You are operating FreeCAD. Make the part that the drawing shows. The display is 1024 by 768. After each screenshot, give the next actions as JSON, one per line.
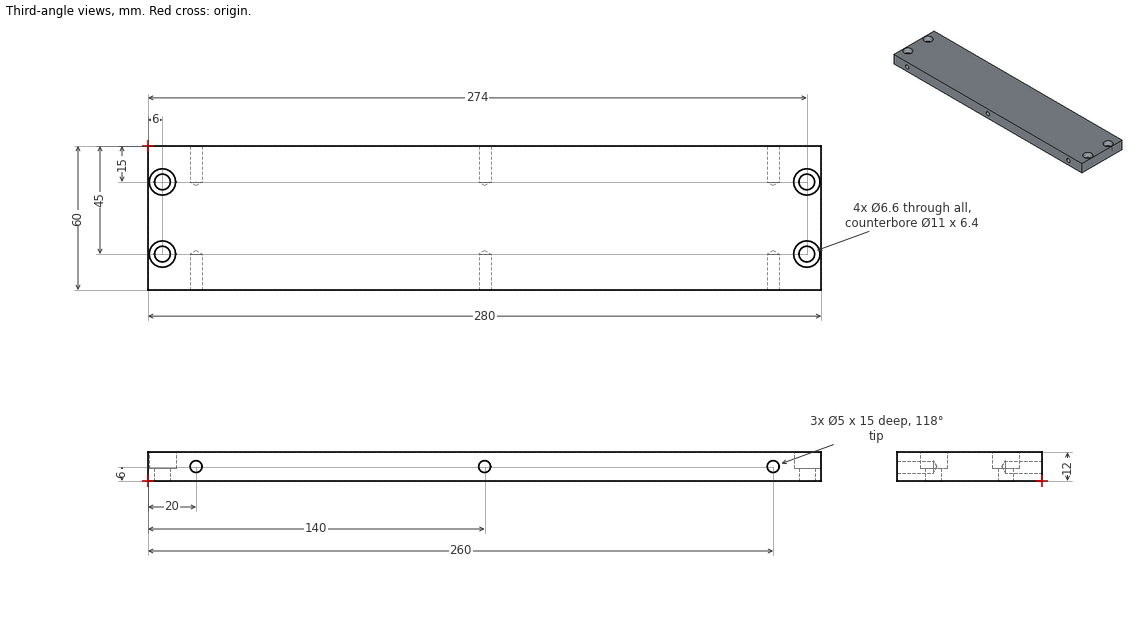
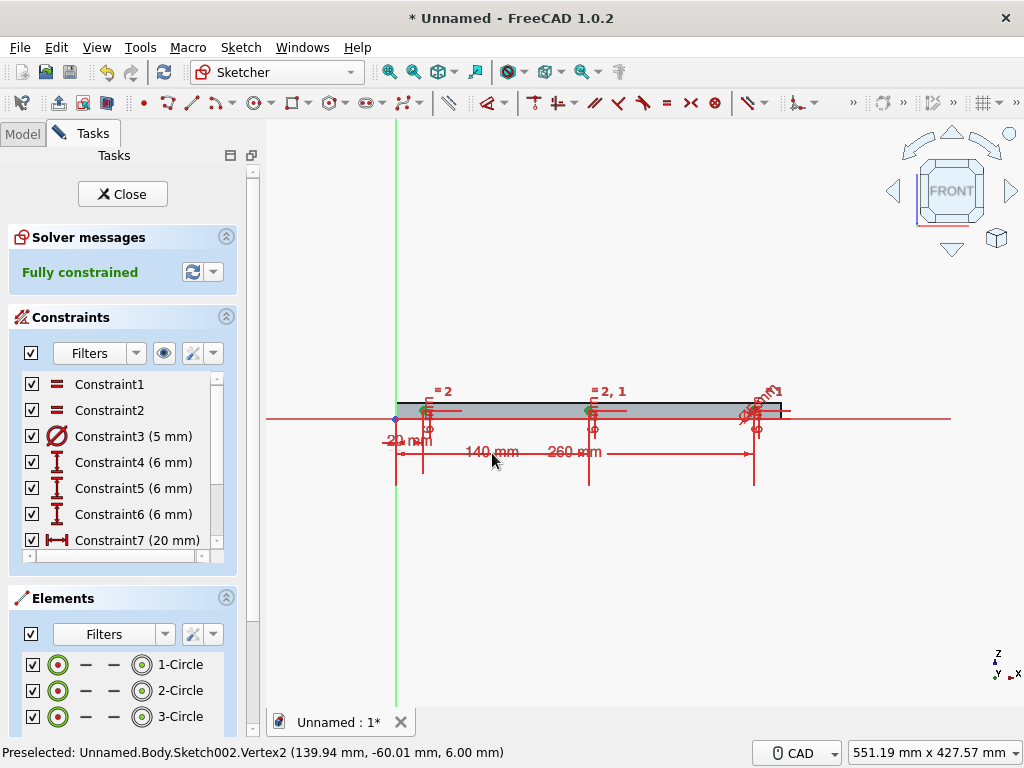
{"action": "left_click", "coordinate": [123, 194]}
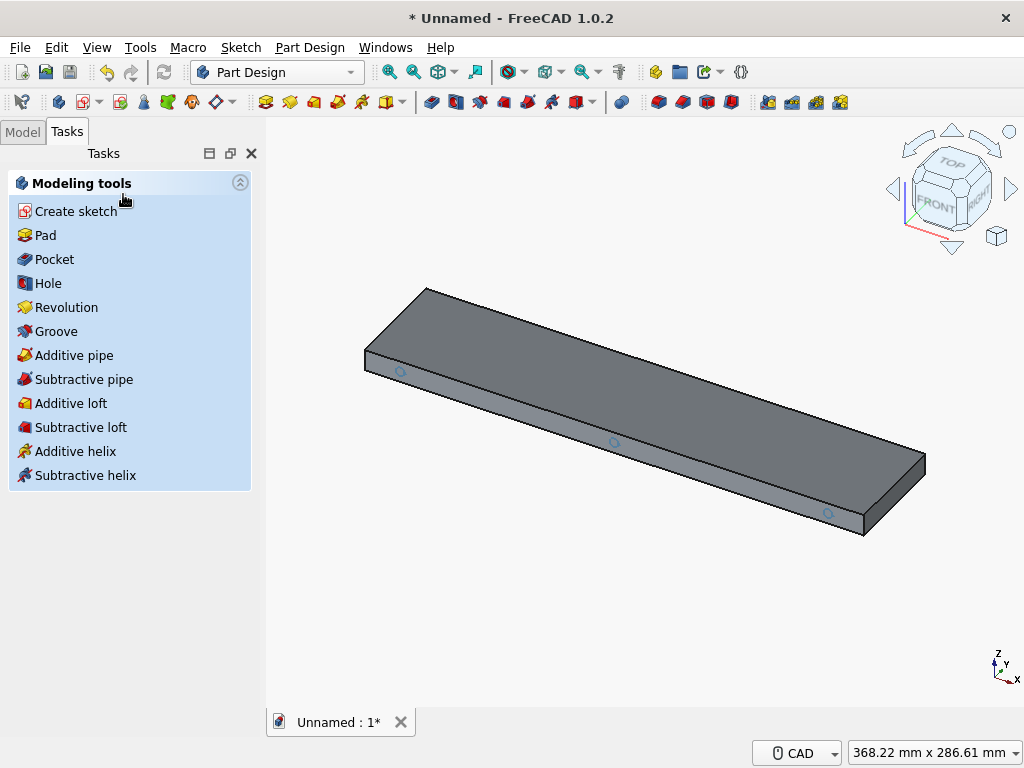
{"action": "left_click", "coordinate": [456, 102]}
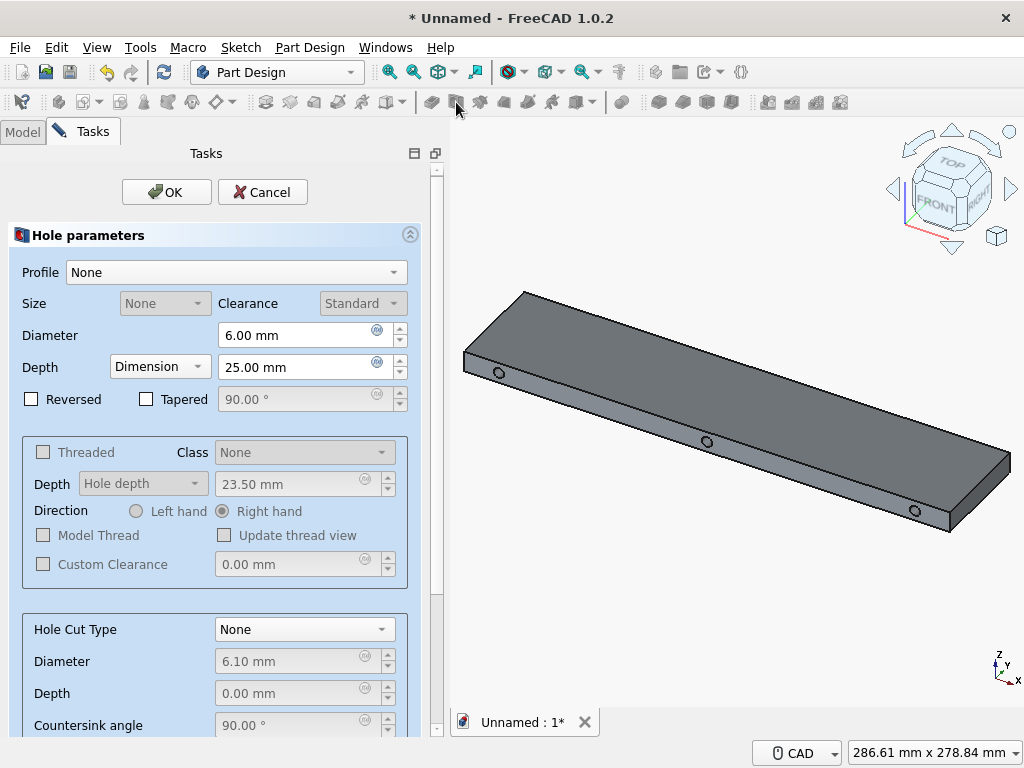
{"action": "triple_click", "coordinate": [305, 335]}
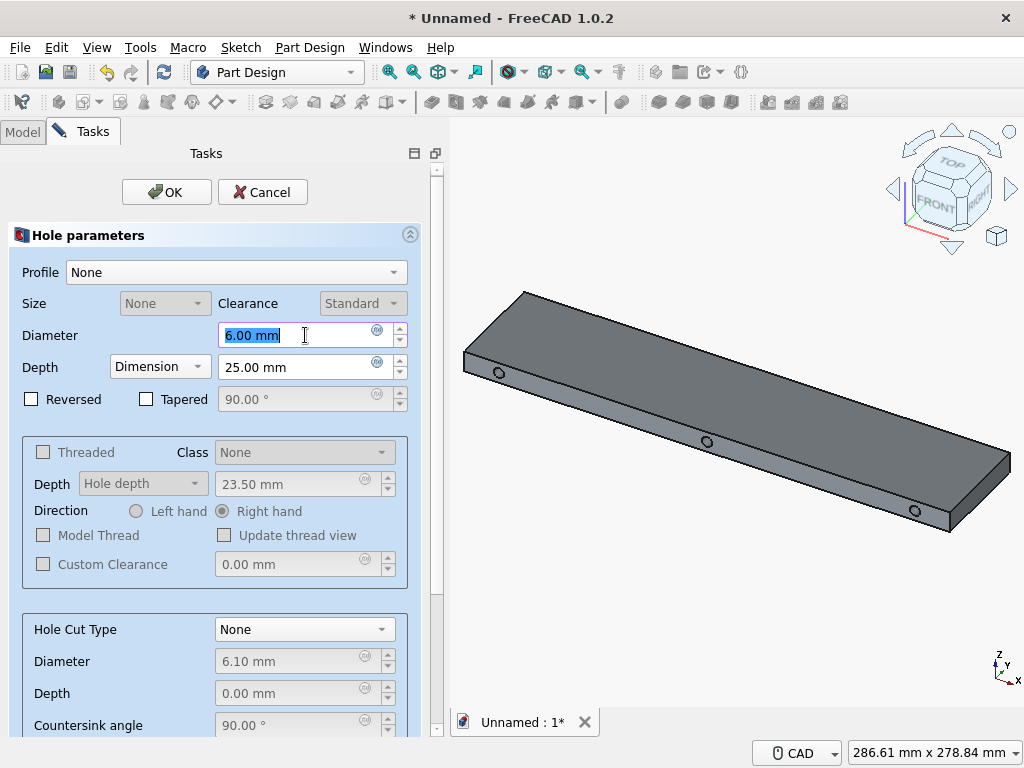
{"action": "type", "text": "5"}
{"action": "key", "text": "Tab"}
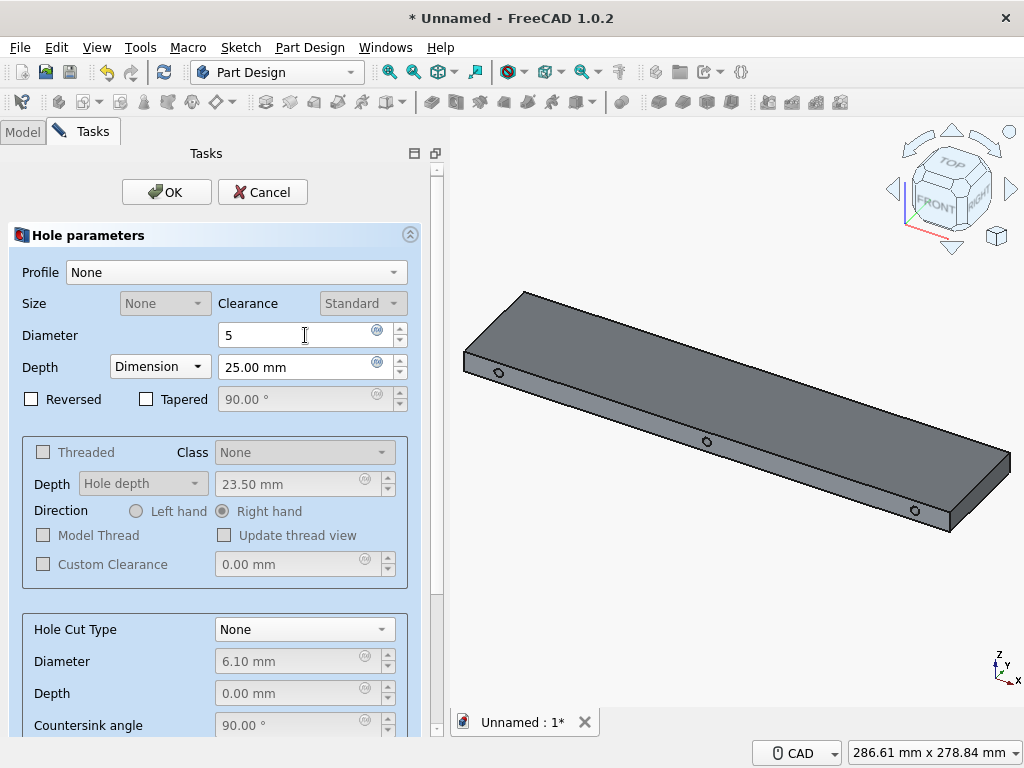
{"action": "triple_click", "coordinate": [305, 367]}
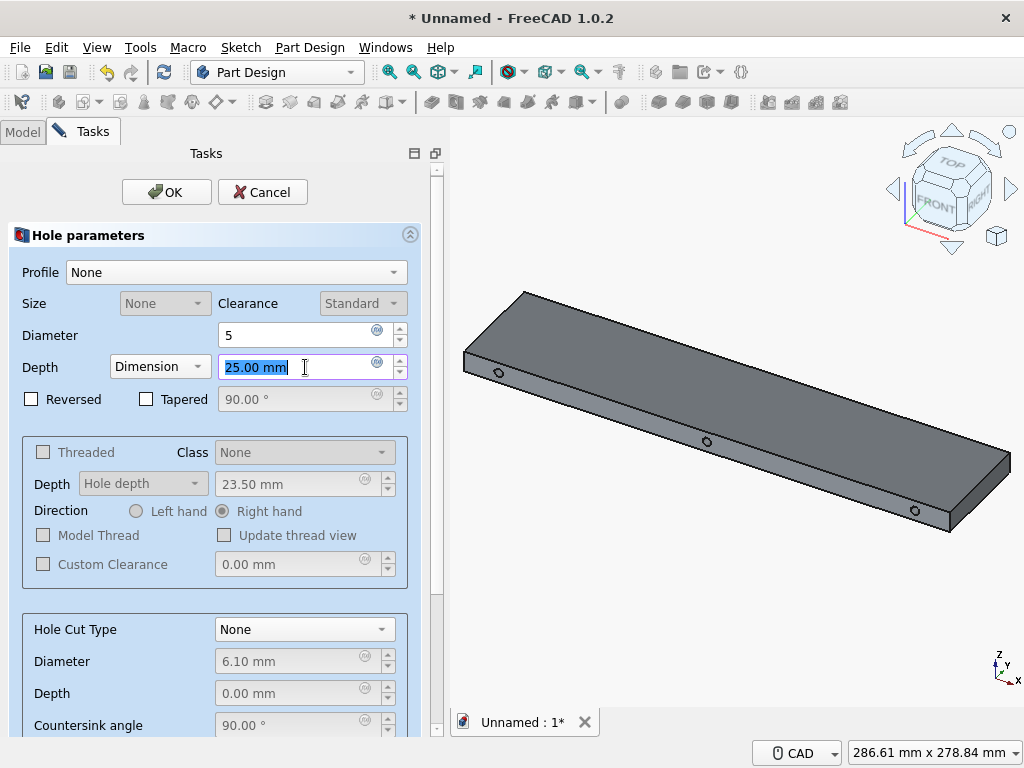
{"action": "type", "text": "15"}
{"action": "key", "text": "Tab"}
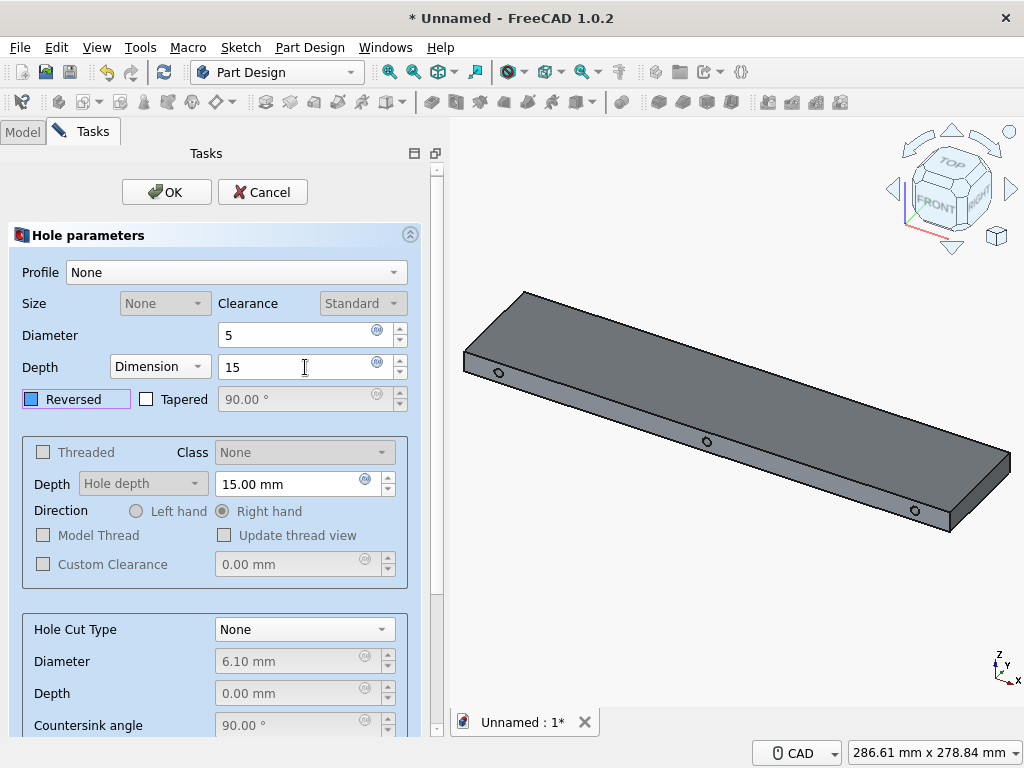
{"action": "left_click", "coordinate": [167, 192]}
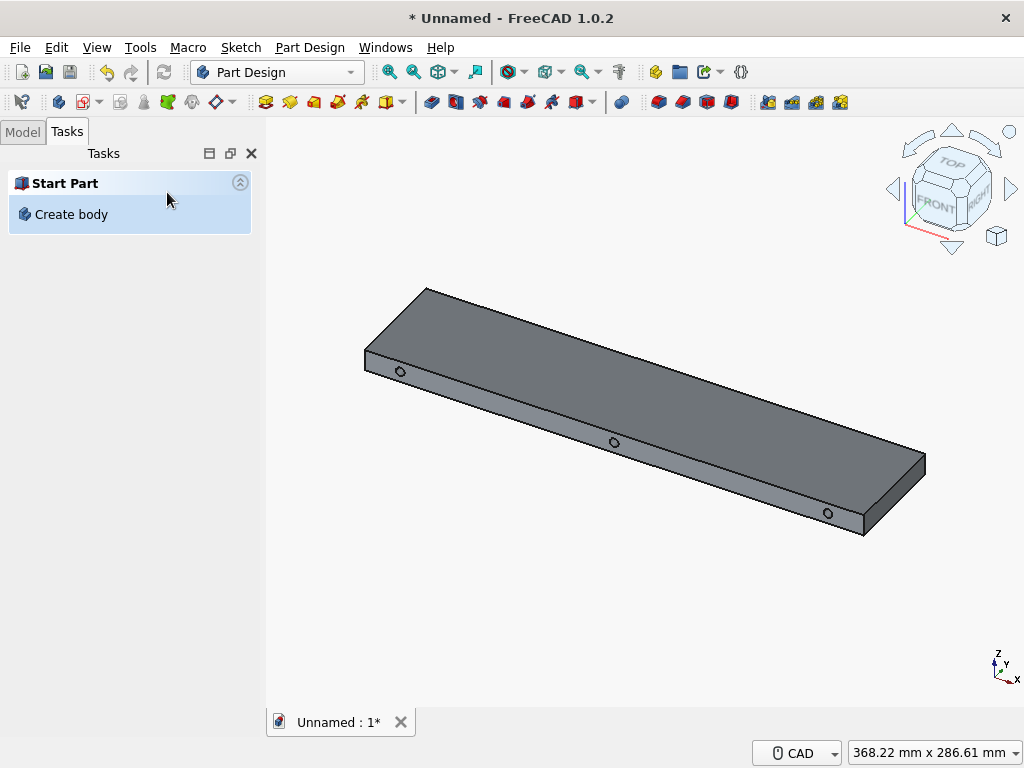
{"action": "left_click", "coordinate": [788, 448]}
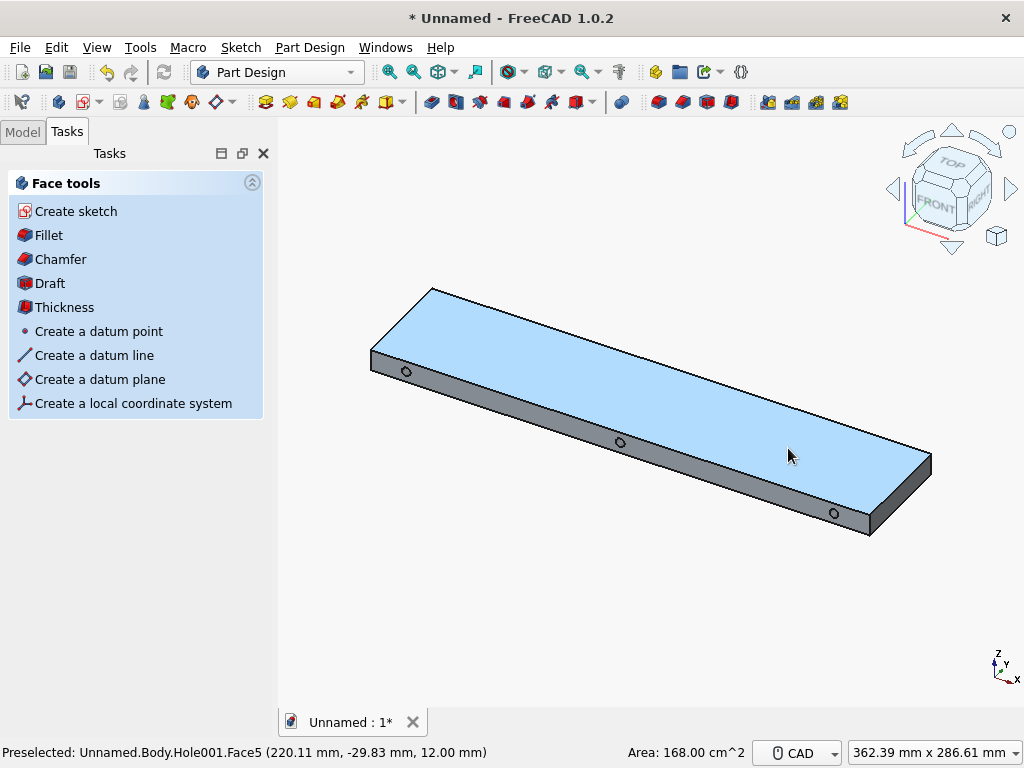
{"action": "left_click", "coordinate": [84, 102]}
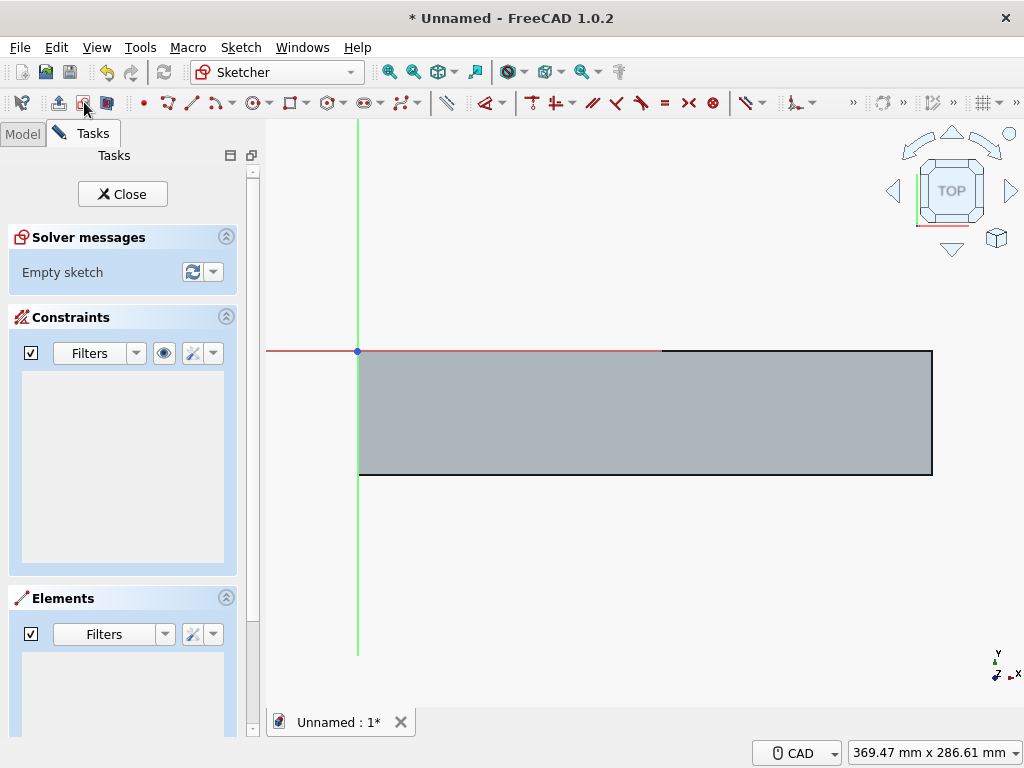
{"action": "scroll", "coordinate": [443, 437], "scroll_direction": "down", "scroll_amount": 2}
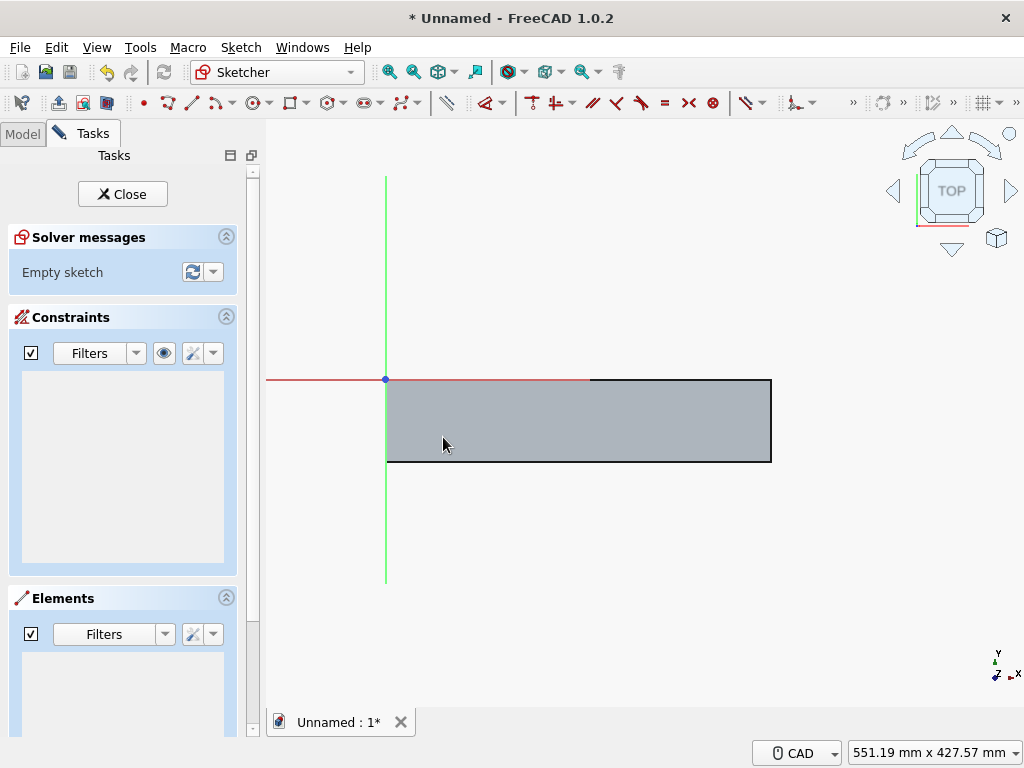
{"action": "left_click", "coordinate": [254, 104]}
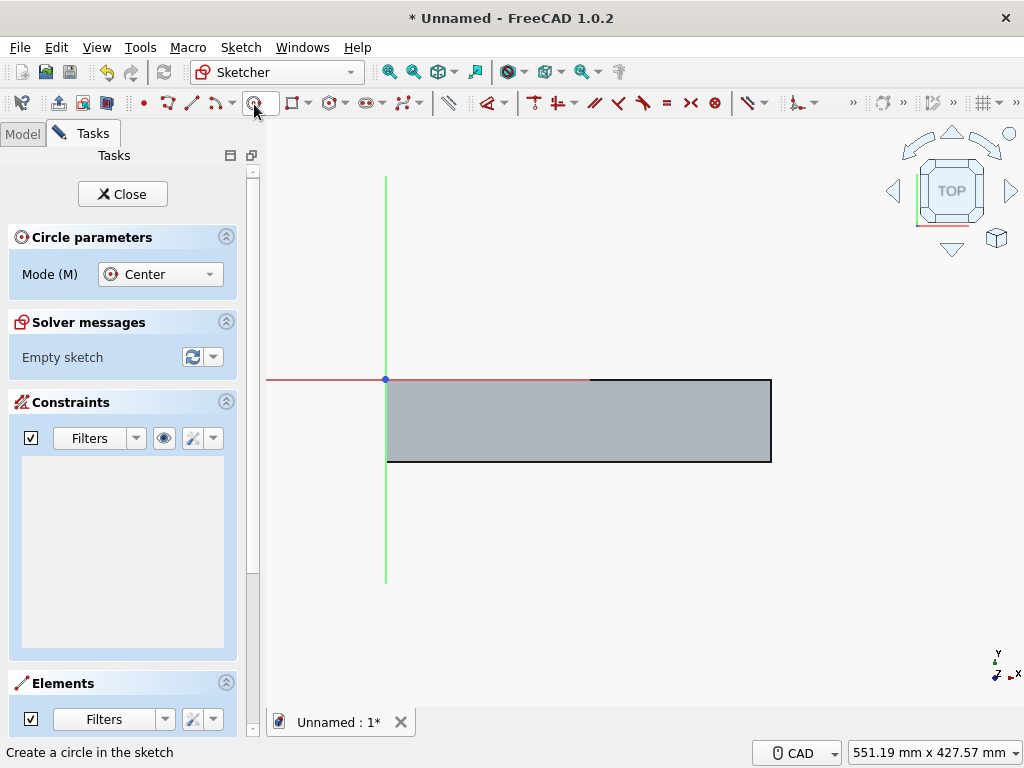
{"action": "scroll", "coordinate": [763, 442], "scroll_direction": "up", "scroll_amount": 9}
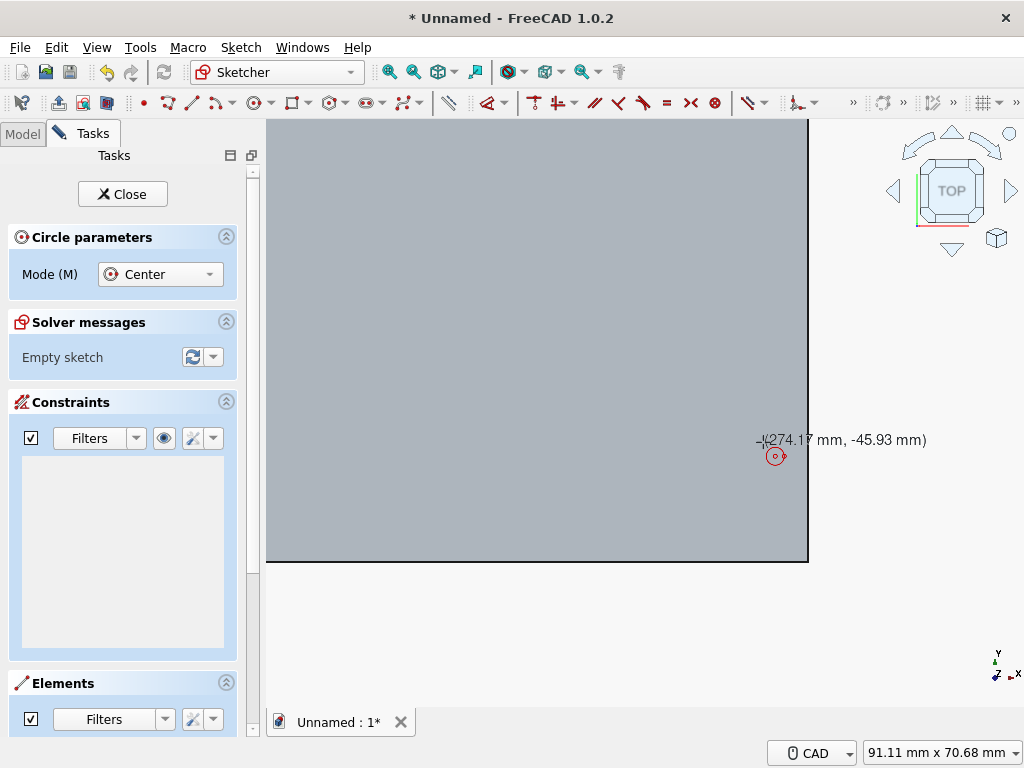
{"action": "scroll", "coordinate": [764, 442], "scroll_direction": "down", "scroll_amount": 9}